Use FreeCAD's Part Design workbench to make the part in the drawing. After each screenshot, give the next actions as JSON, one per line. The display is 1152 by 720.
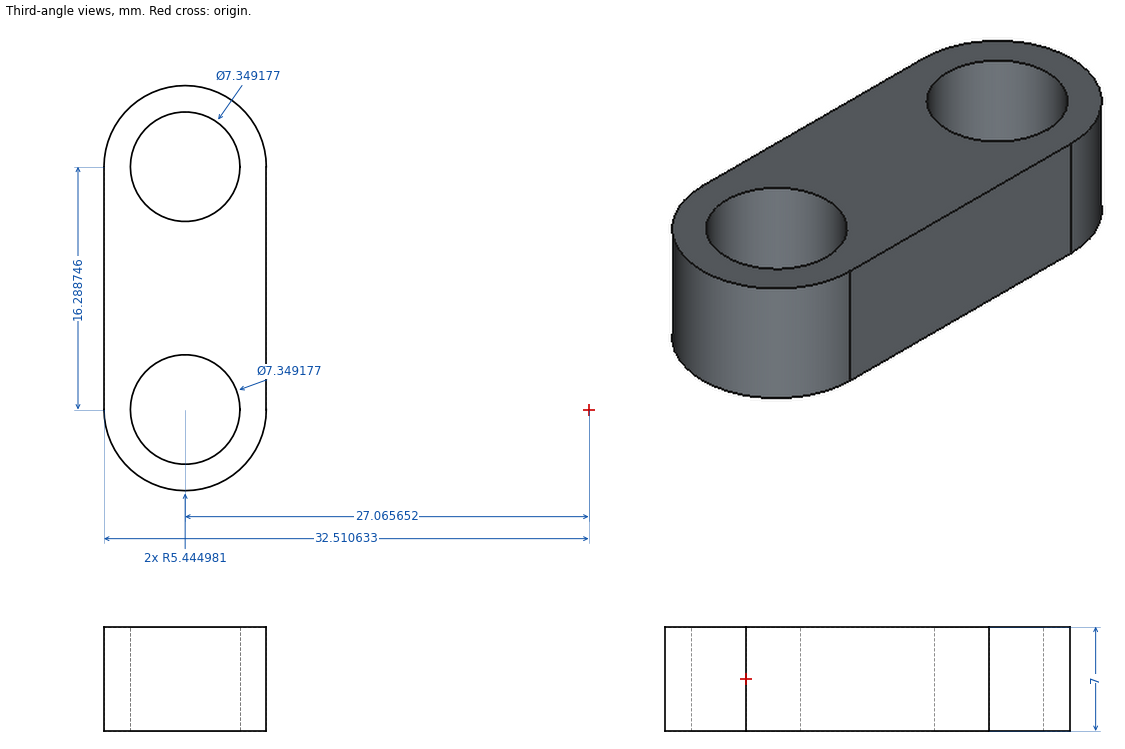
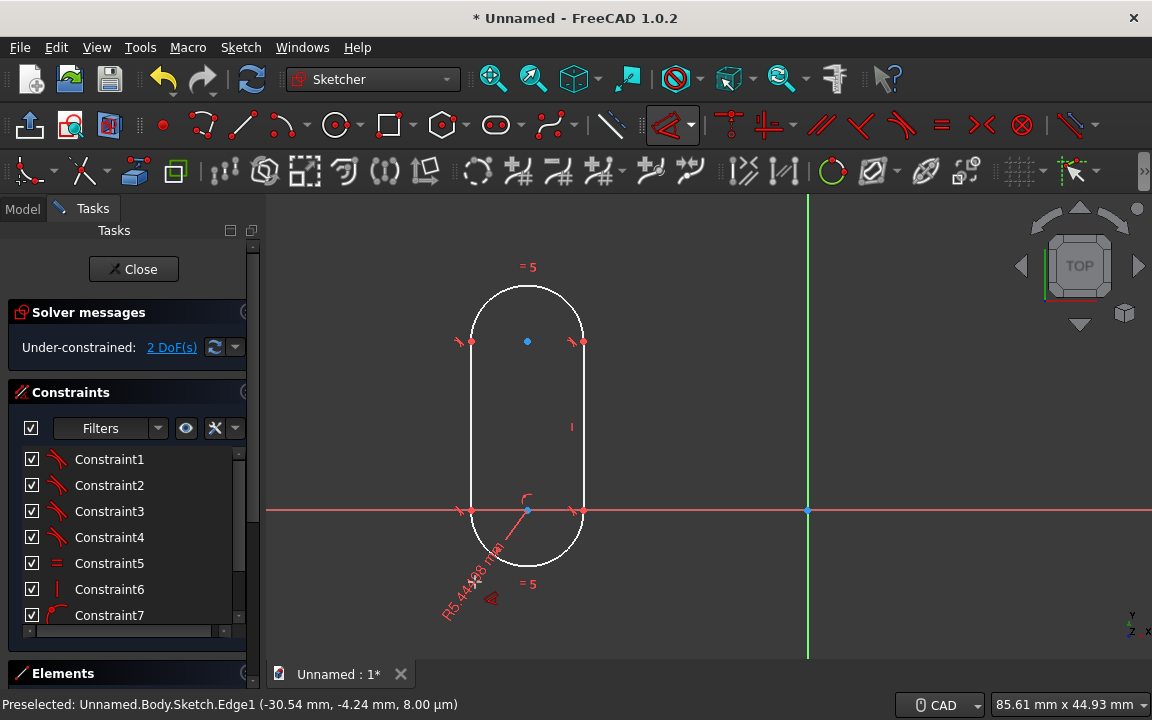
{"action": "left_click", "coordinate": [471, 460]}
{"action": "left_click", "coordinate": [437, 426]}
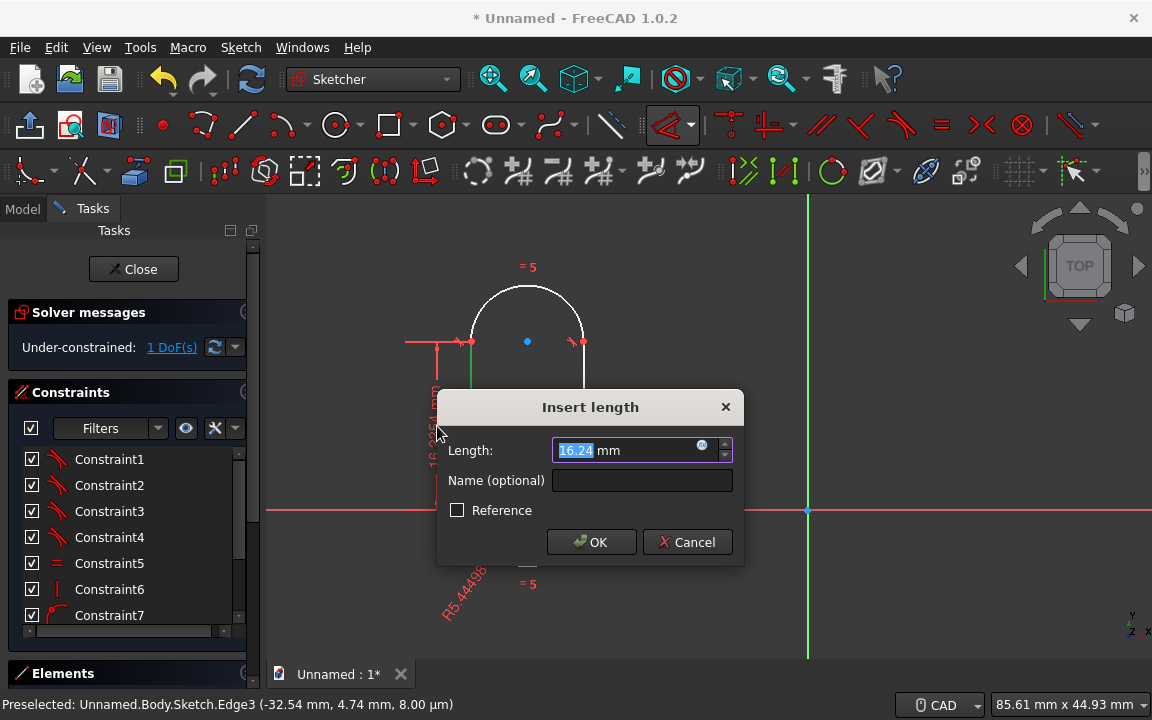
{"action": "type", "text": "16.288746"}
{"action": "key", "text": "Return"}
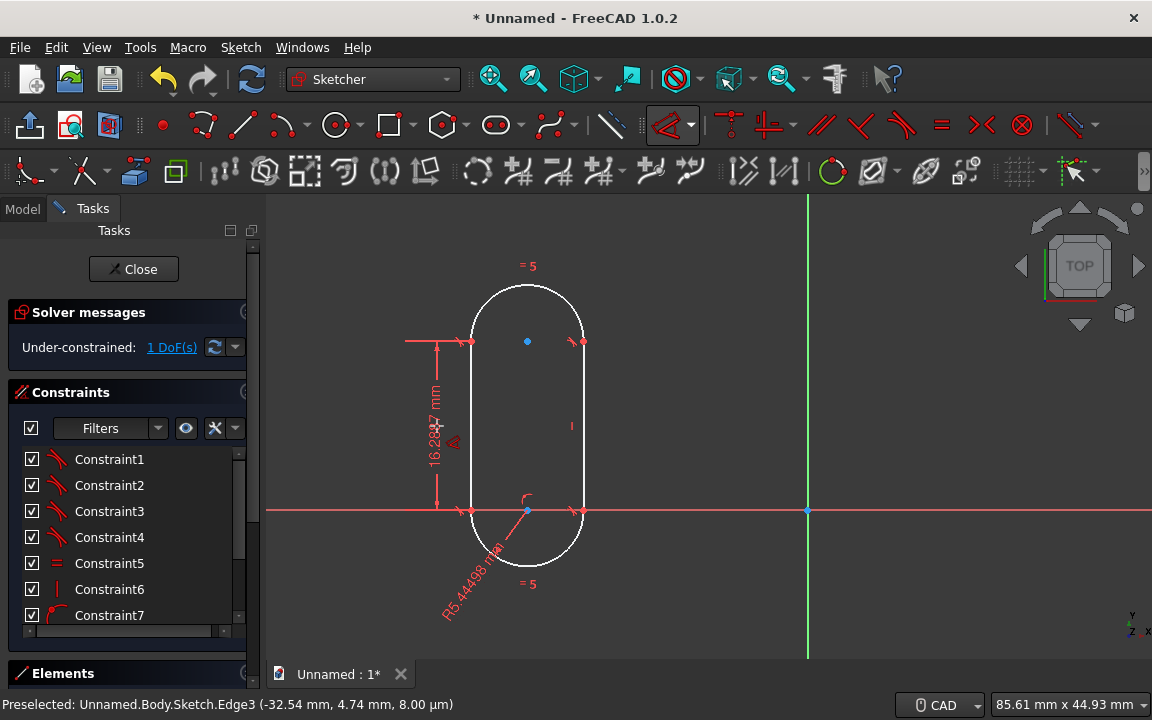
{"action": "left_click", "coordinate": [471, 510]}
{"action": "left_click", "coordinate": [639, 544]}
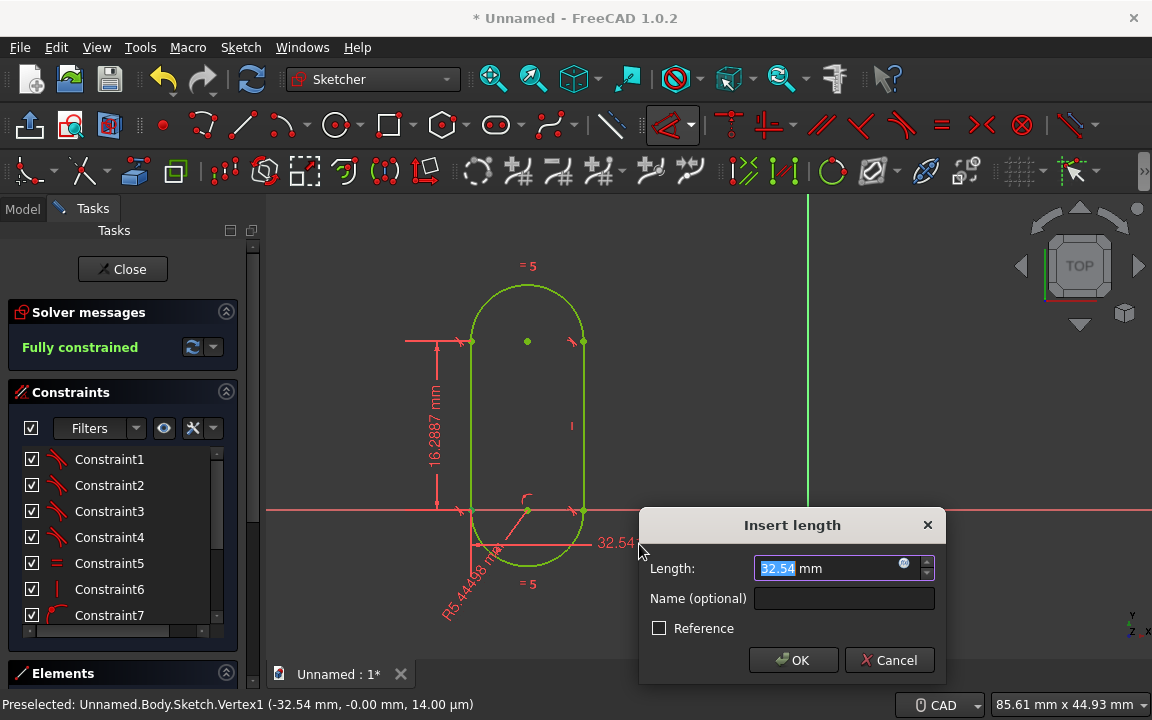
{"action": "type", "text": "32.510633"}
{"action": "key", "text": "Return"}
{"action": "key", "text": "Escape"}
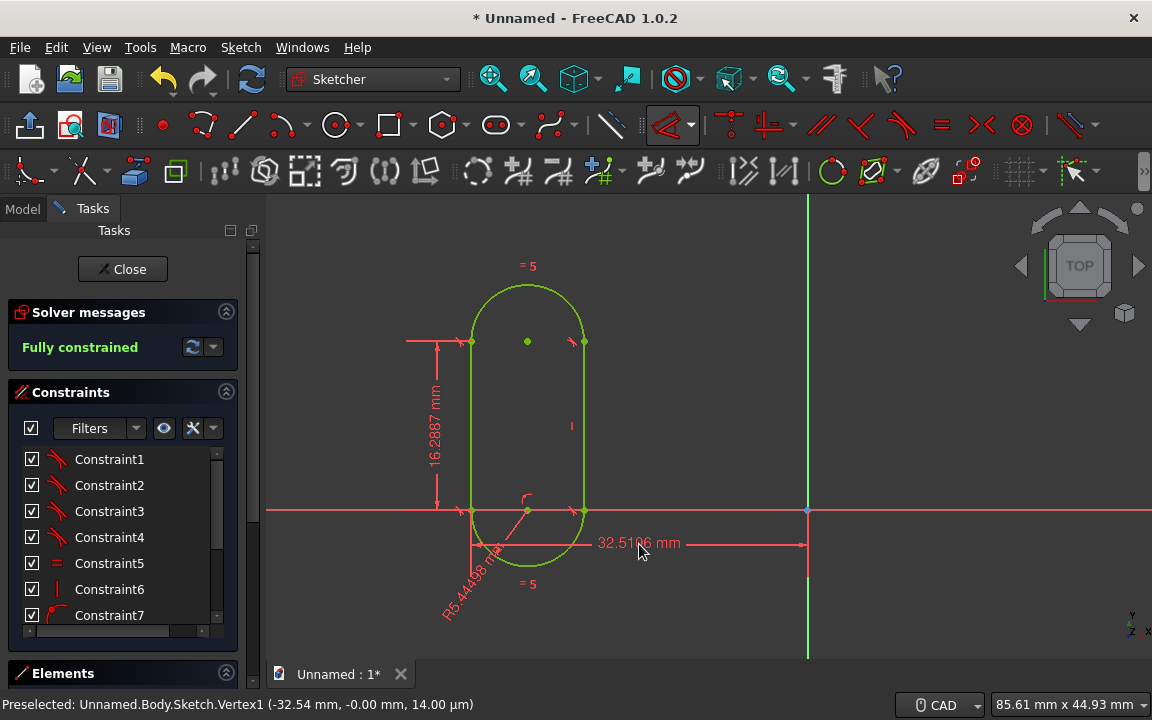
{"action": "left_click", "coordinate": [123, 269]}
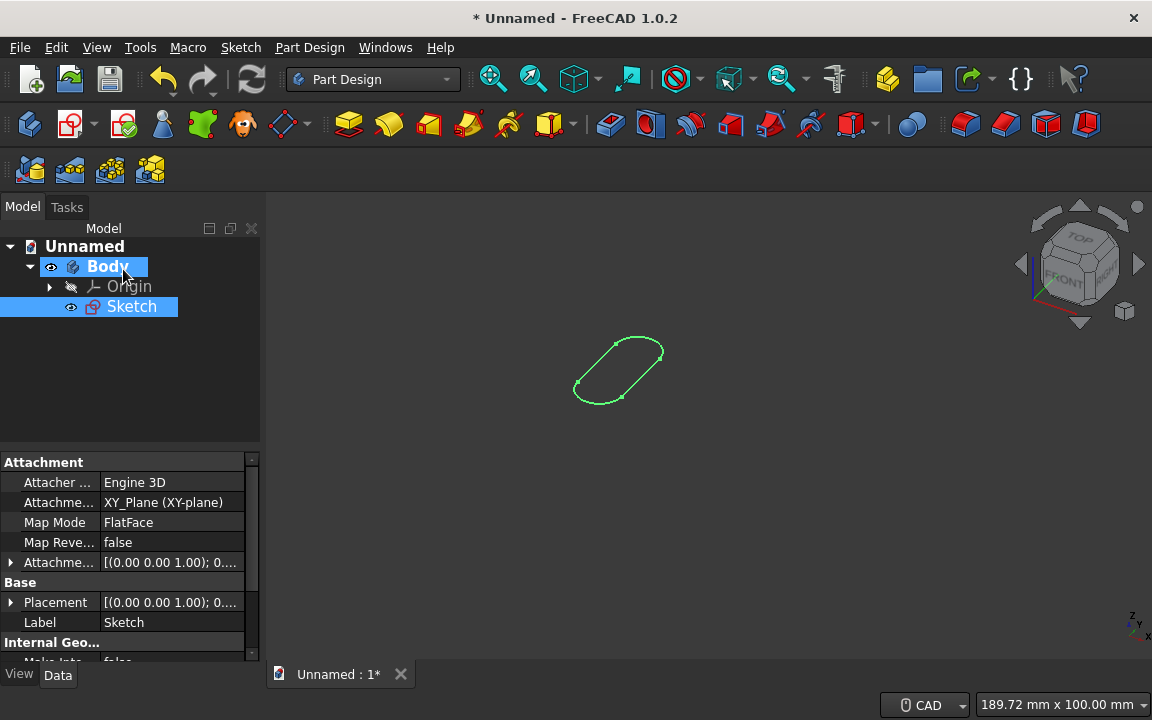
{"action": "left_click", "coordinate": [350, 124]}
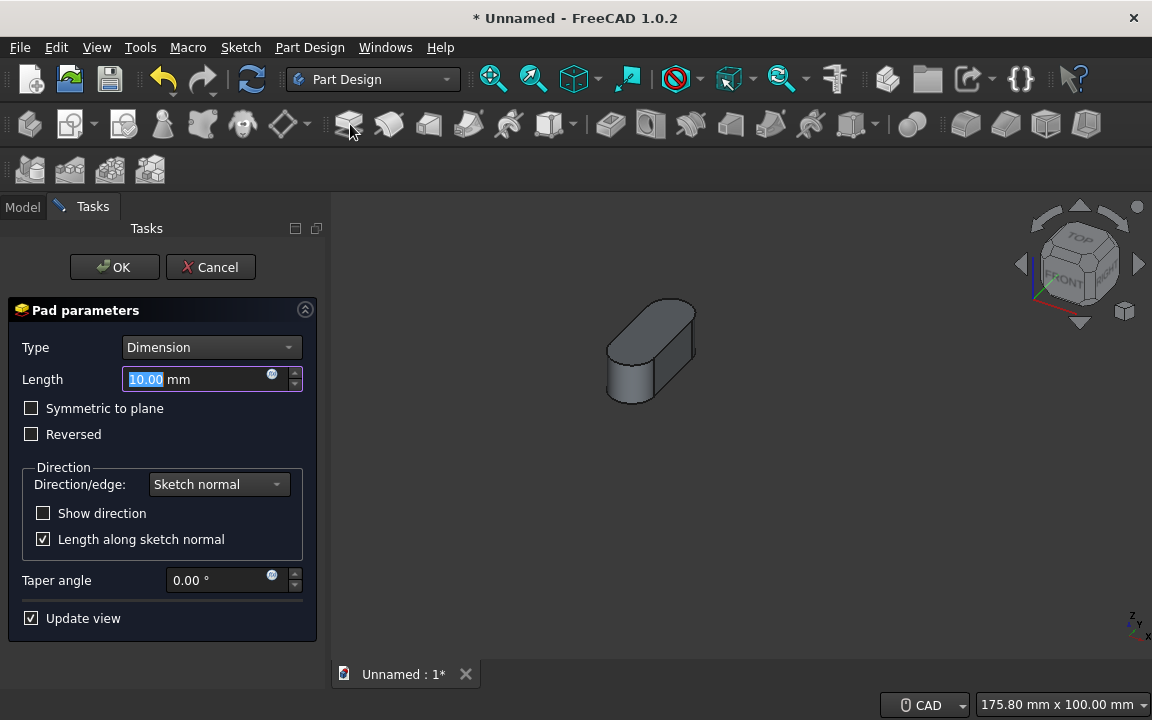
{"action": "type", "text": "7"}
{"action": "key", "text": "Tab"}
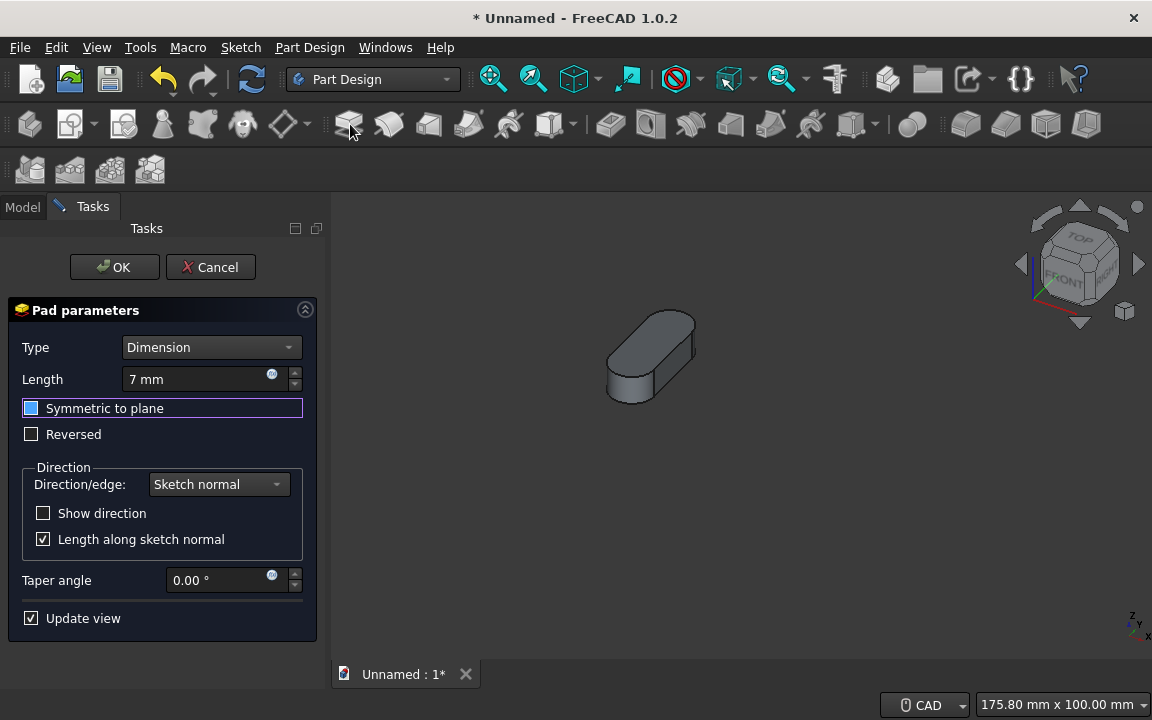
{"action": "left_click", "coordinate": [30, 408]}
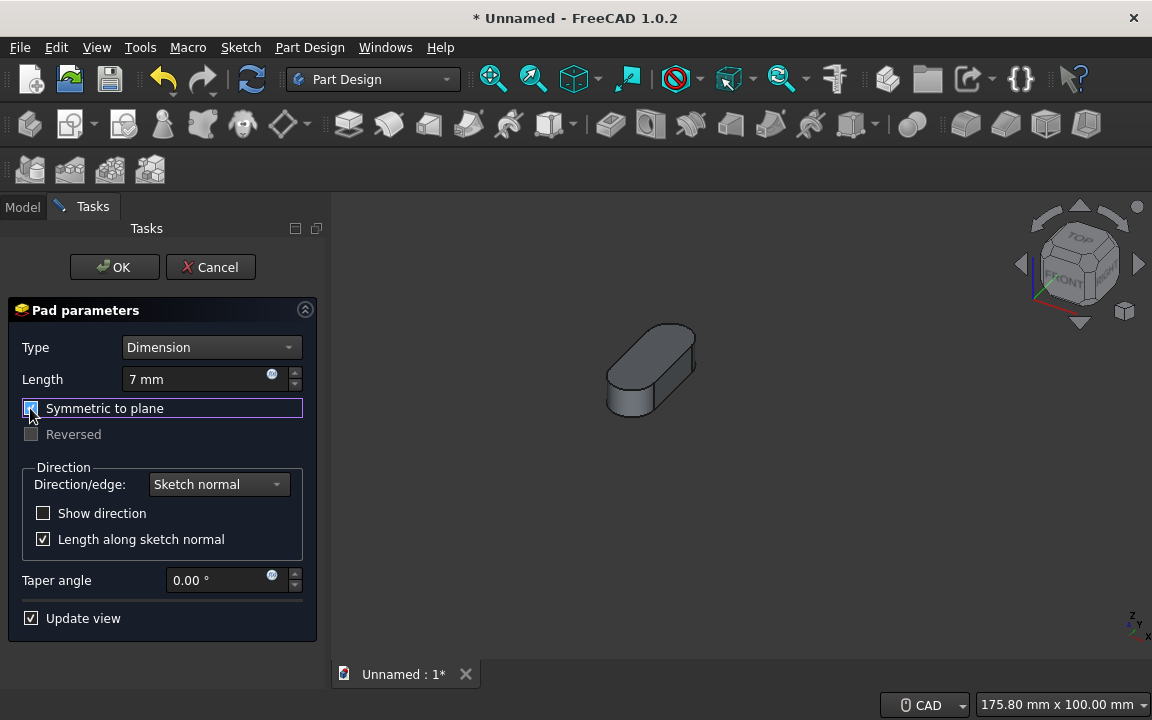
{"action": "left_click", "coordinate": [115, 267]}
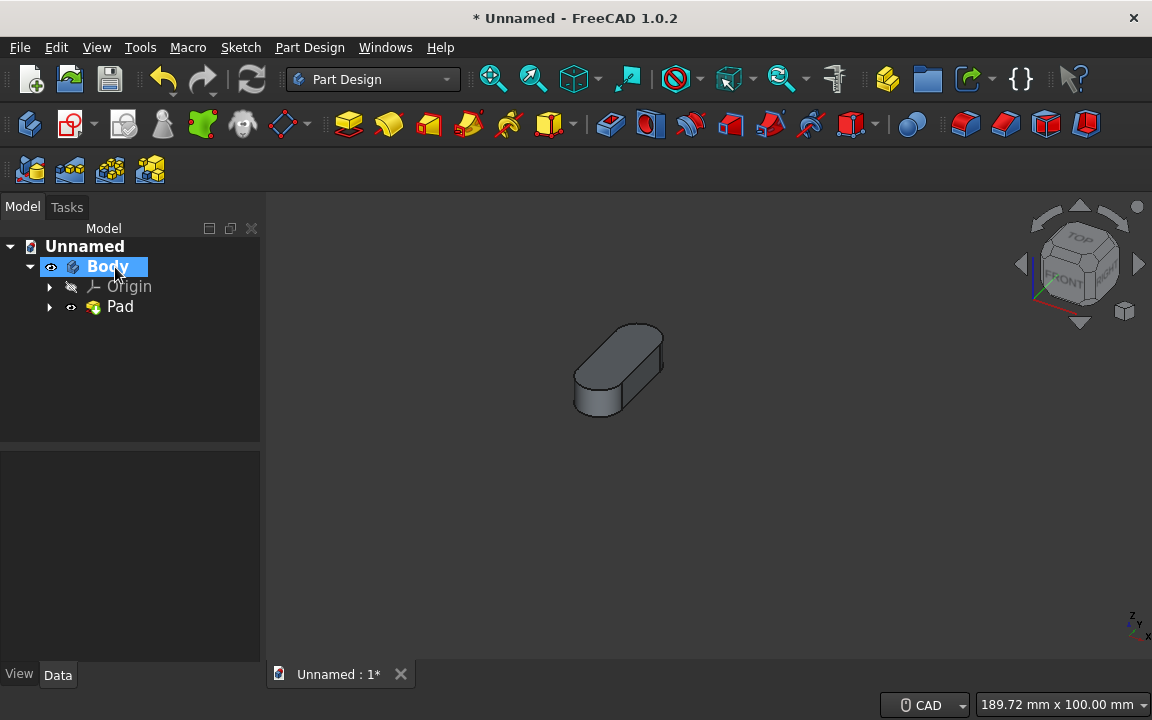
{"action": "left_click", "coordinate": [494, 80]}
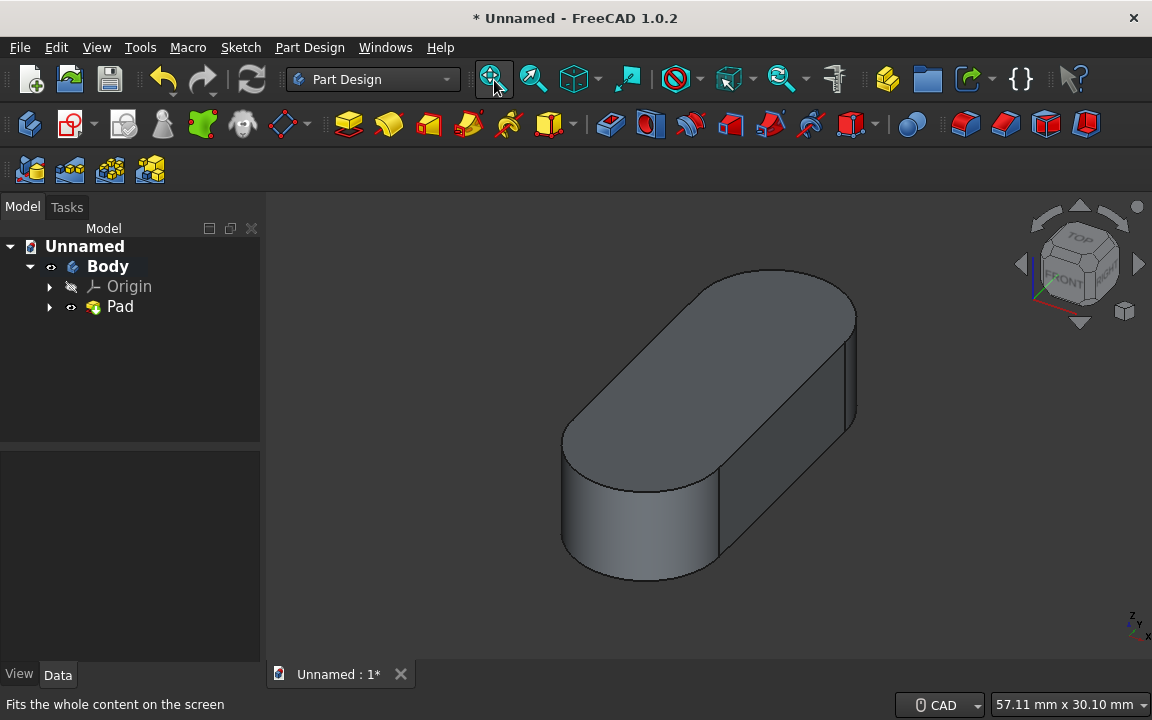
{"action": "left_click", "coordinate": [769, 320]}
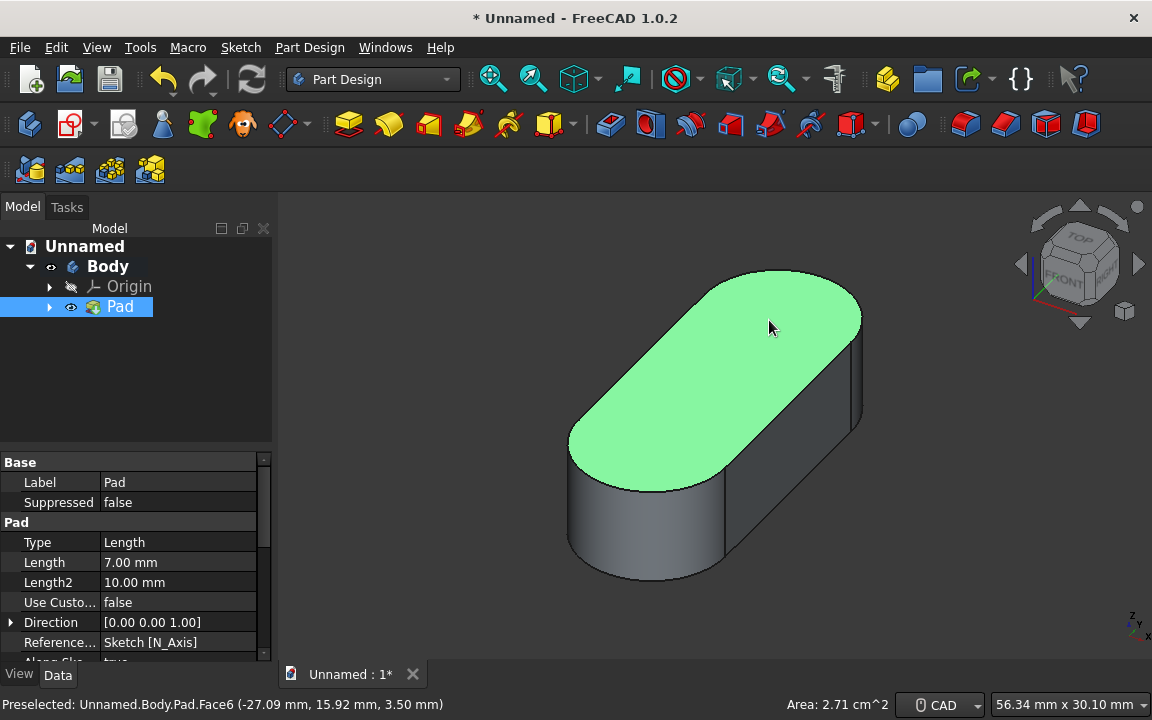
{"action": "left_click", "coordinate": [70, 124]}